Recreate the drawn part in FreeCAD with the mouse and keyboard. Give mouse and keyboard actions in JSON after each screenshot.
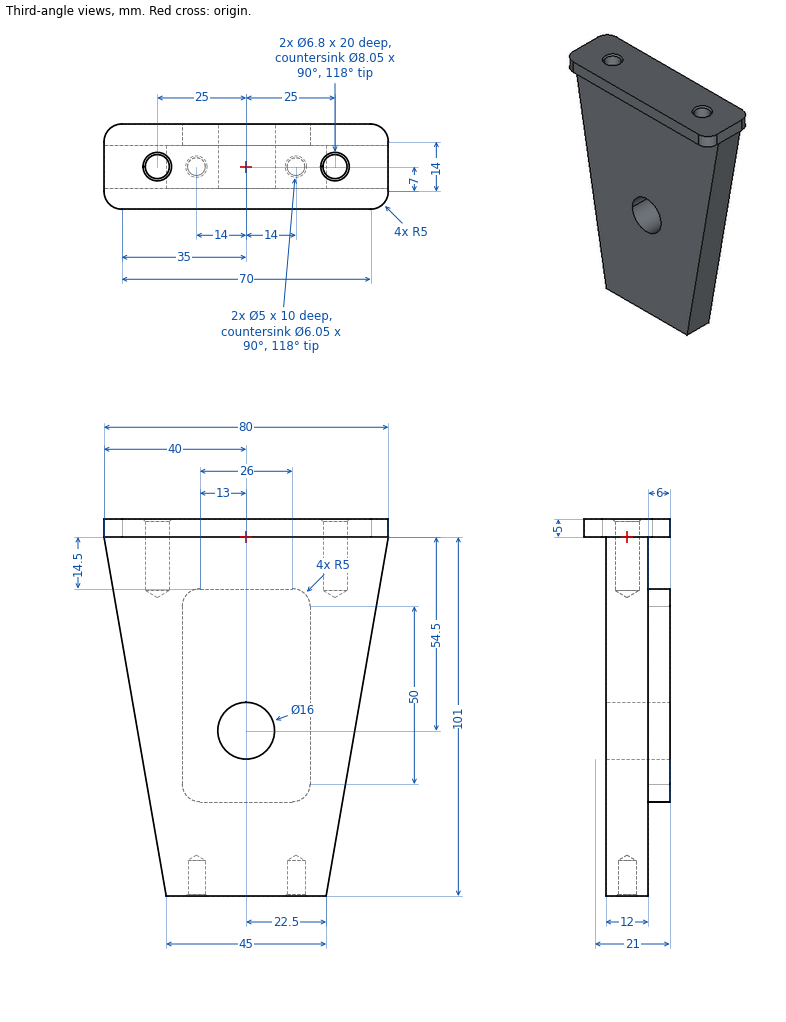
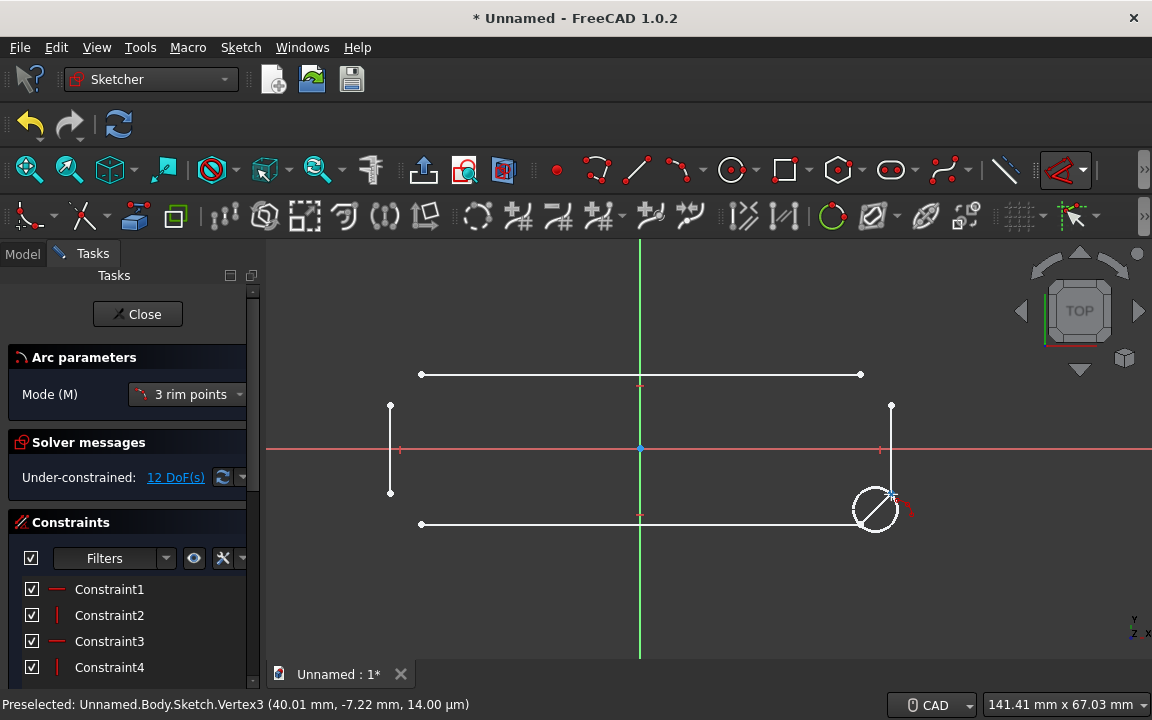
{"action": "scroll", "coordinate": [882, 515], "scroll_direction": "up", "scroll_amount": 3}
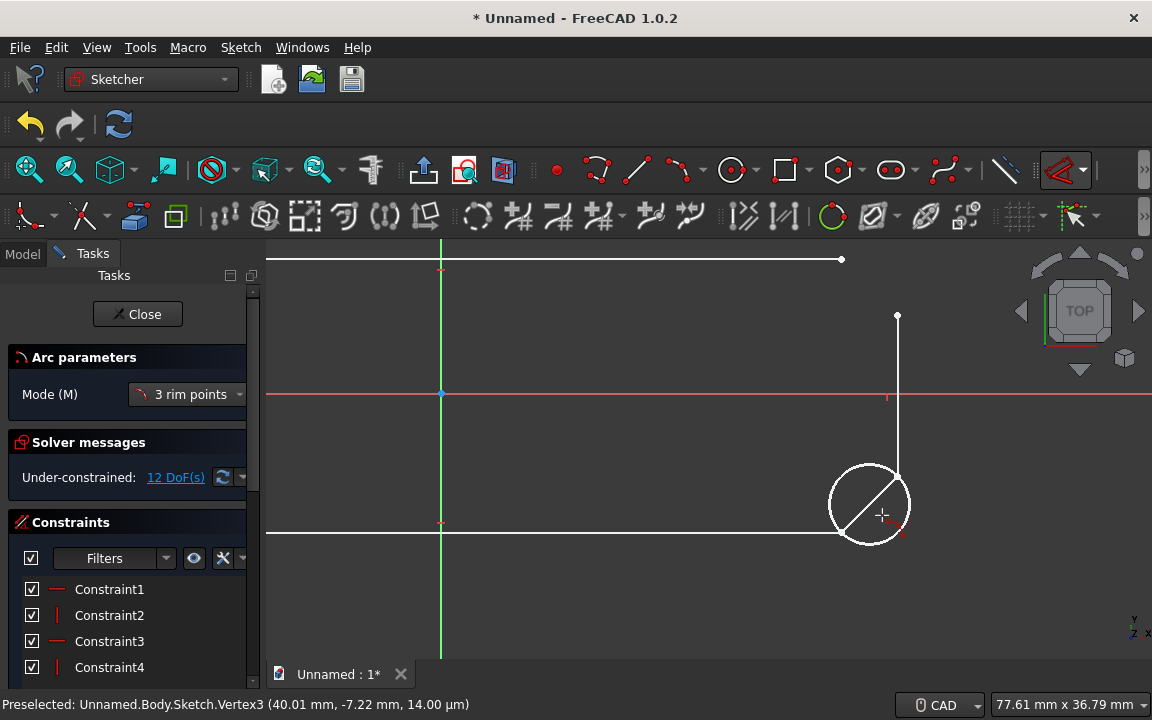
{"action": "left_click", "coordinate": [881, 514]}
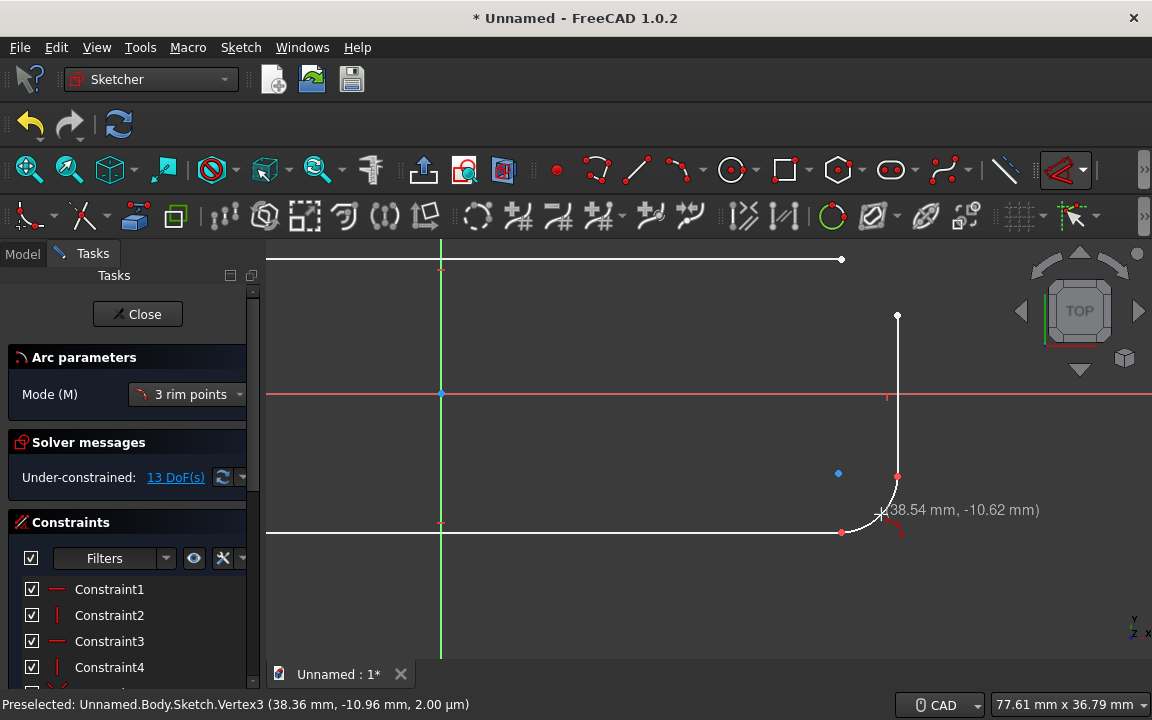
{"action": "left_click", "coordinate": [898, 316]}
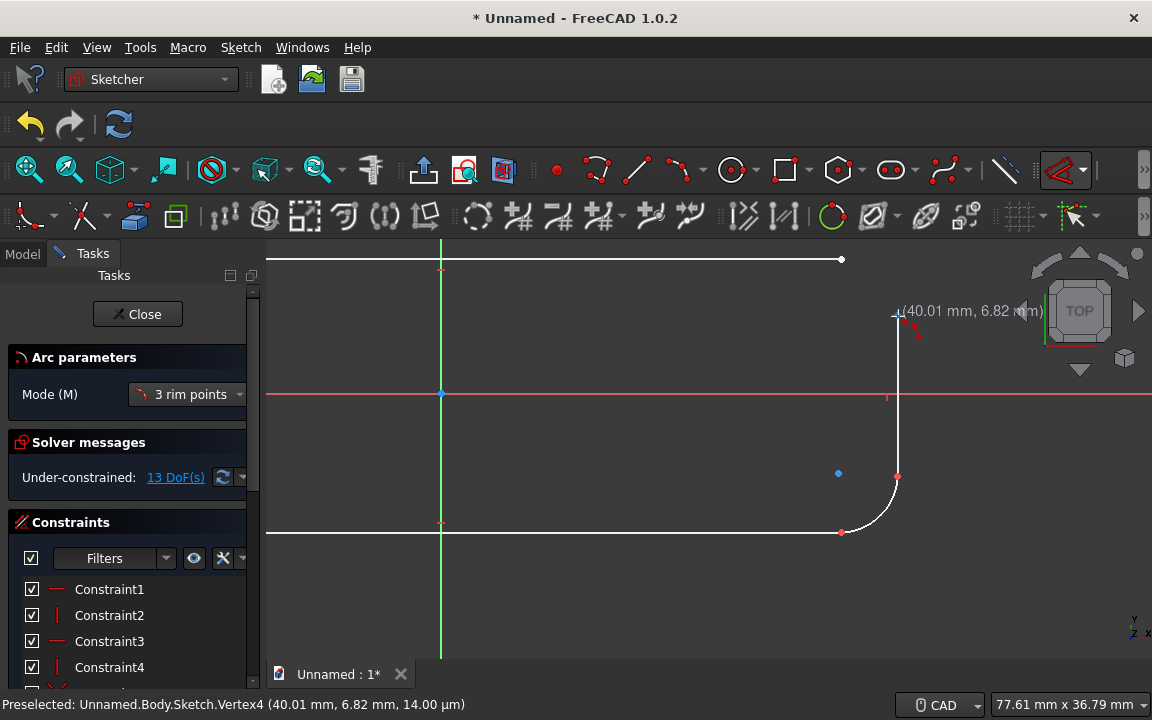
{"action": "scroll", "coordinate": [883, 516], "scroll_direction": "down", "scroll_amount": 3}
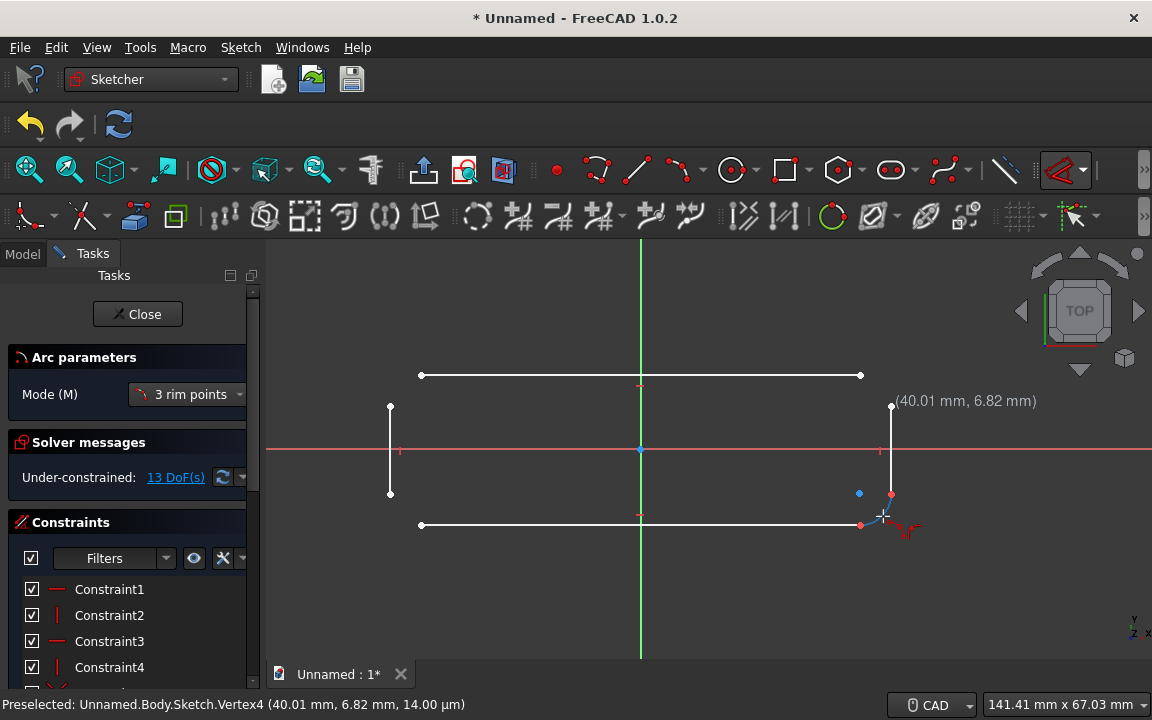
{"action": "left_click", "coordinate": [860, 375]}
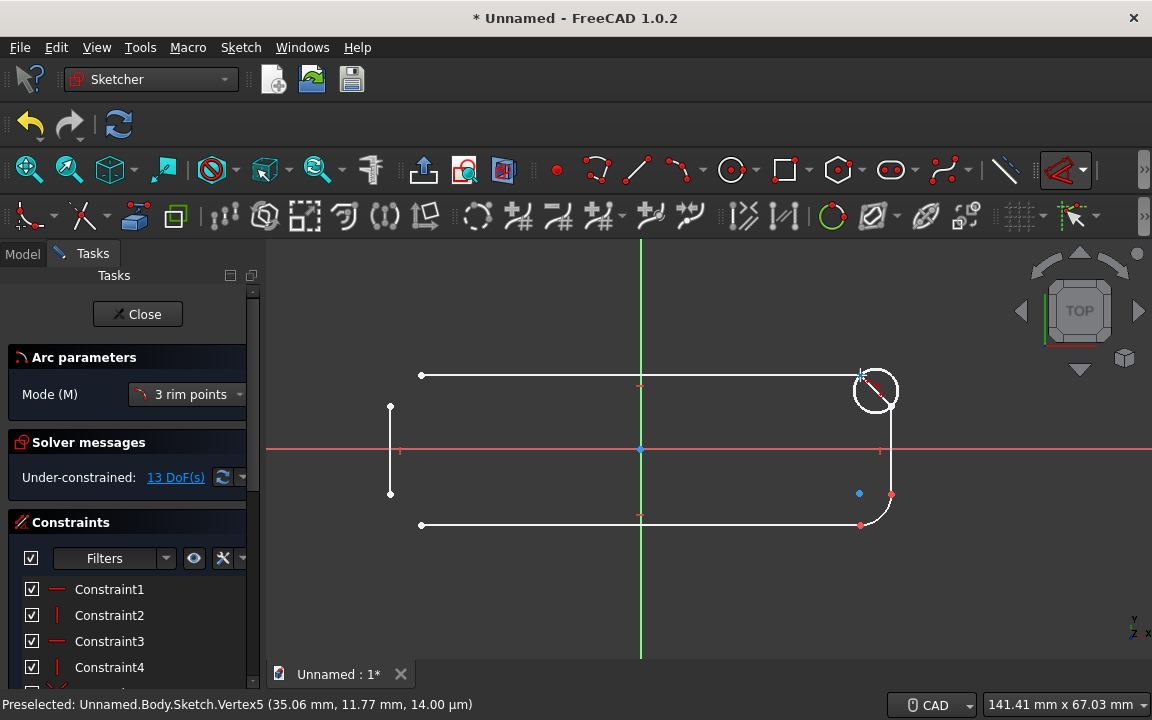
{"action": "scroll", "coordinate": [882, 383], "scroll_direction": "up", "scroll_amount": 3}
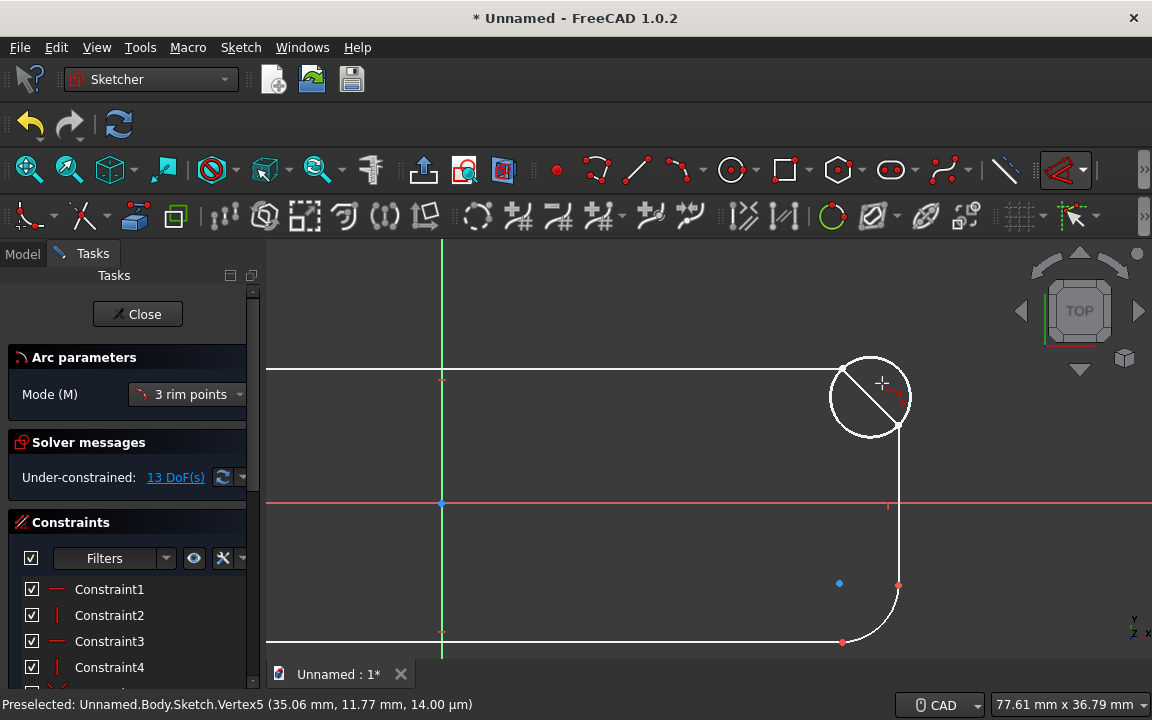
{"action": "left_click", "coordinate": [882, 383]}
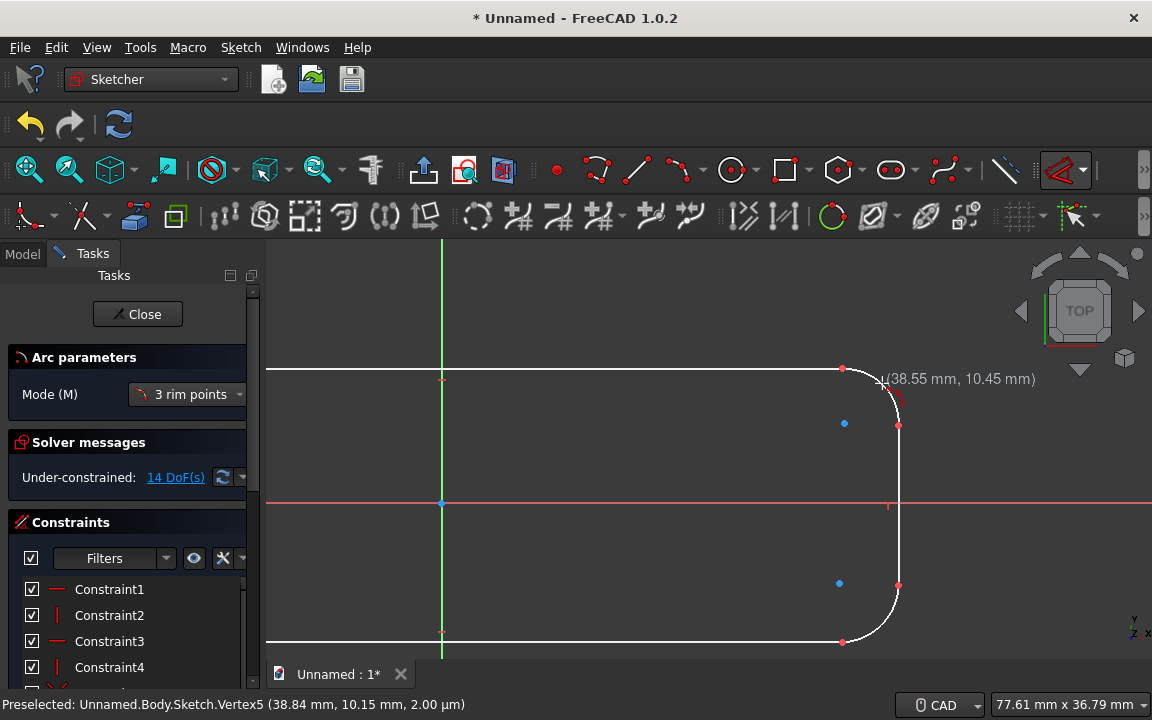
{"action": "scroll", "coordinate": [882, 383], "scroll_direction": "down", "scroll_amount": 3}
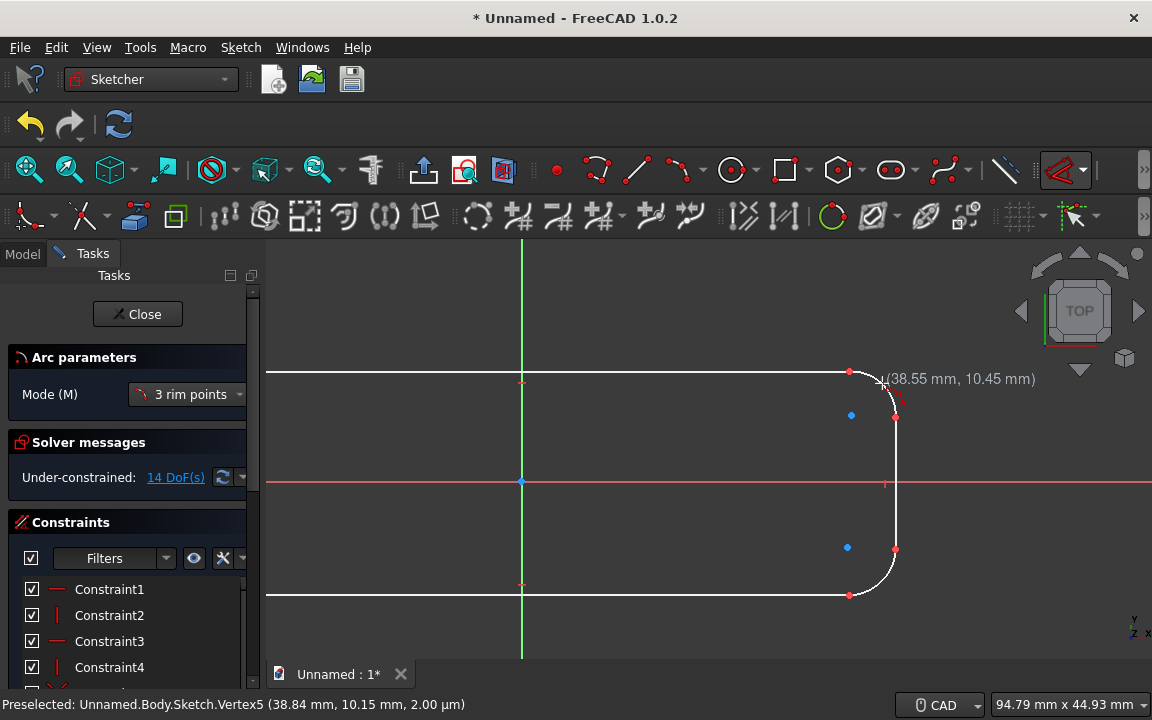
{"action": "left_click", "coordinate": [421, 375]}
{"action": "left_click", "coordinate": [390, 406]}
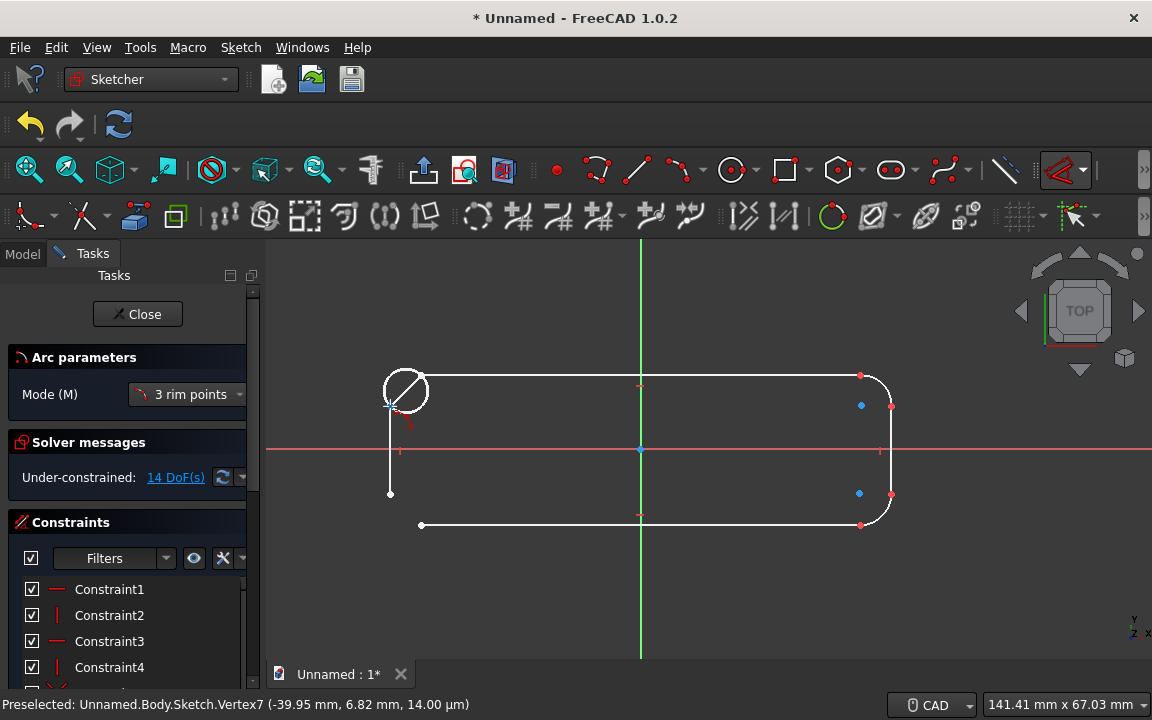
{"action": "scroll", "coordinate": [399, 383], "scroll_direction": "up", "scroll_amount": 3}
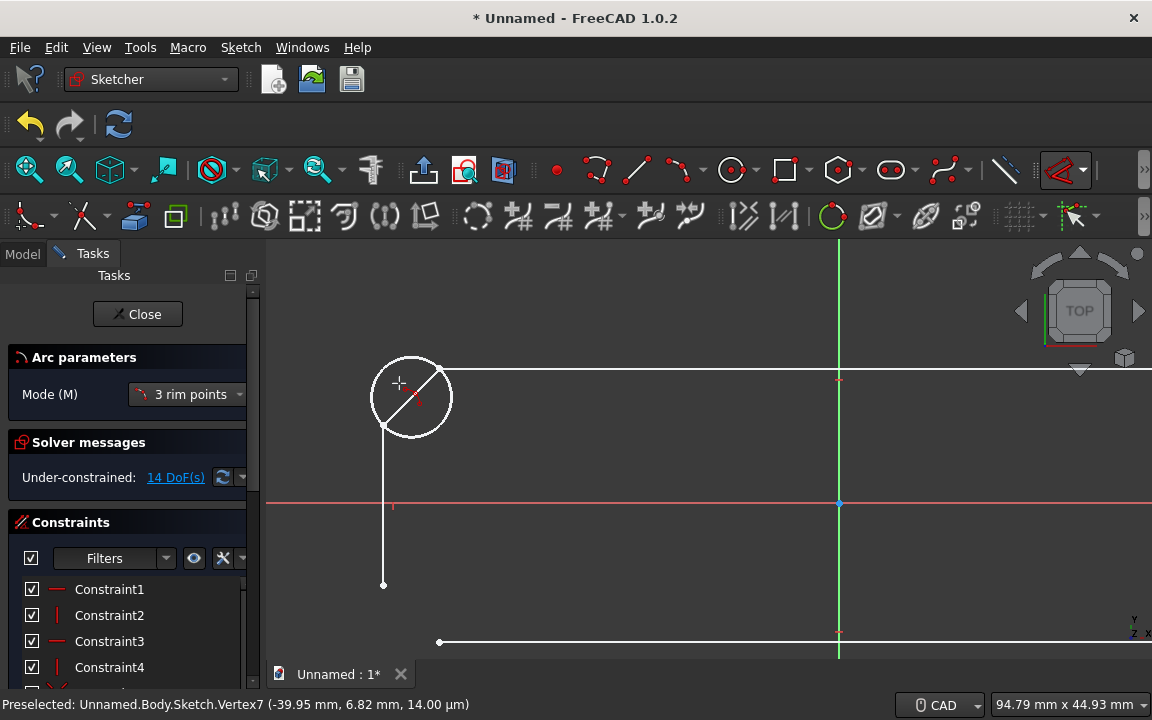
{"action": "left_click", "coordinate": [399, 383]}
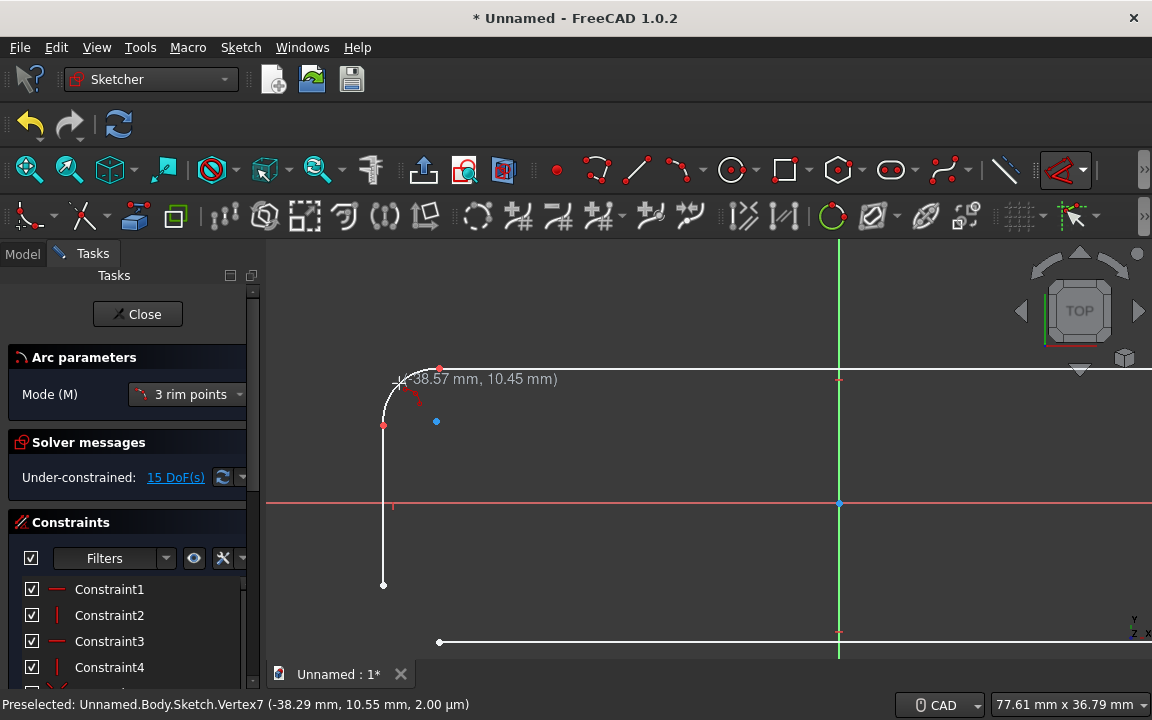
{"action": "left_click", "coordinate": [383, 586]}